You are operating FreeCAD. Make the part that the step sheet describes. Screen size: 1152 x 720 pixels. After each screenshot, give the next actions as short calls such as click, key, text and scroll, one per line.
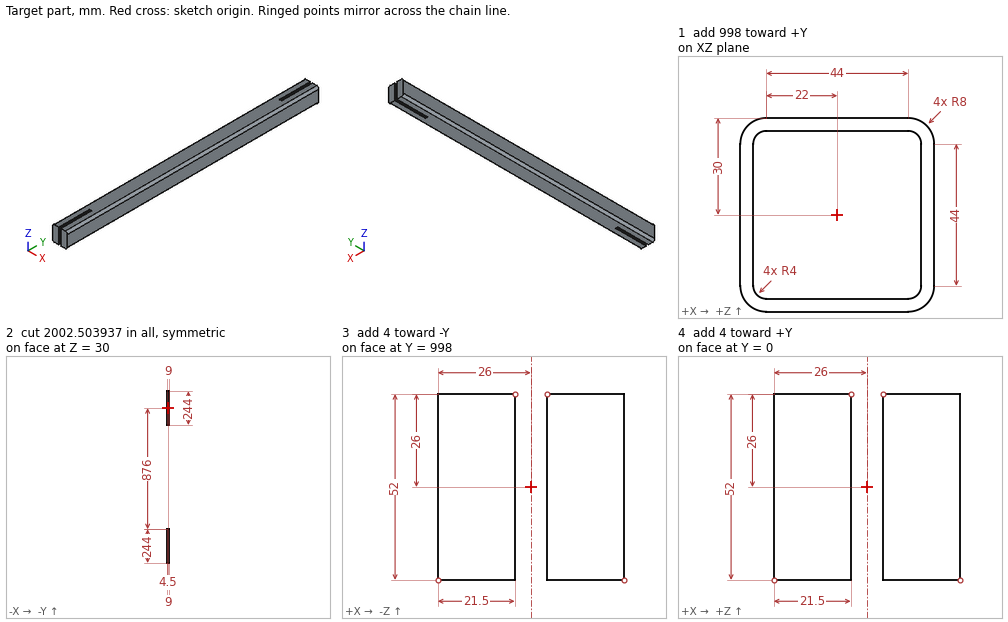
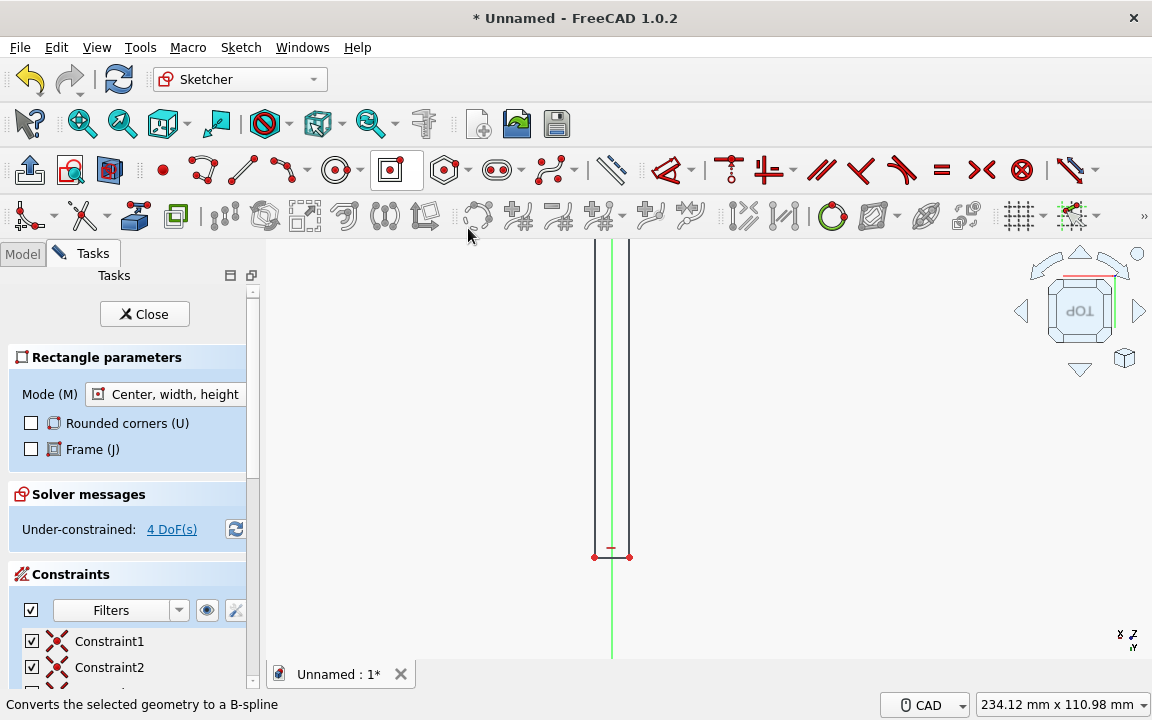
scroll(642, 566, down, 15)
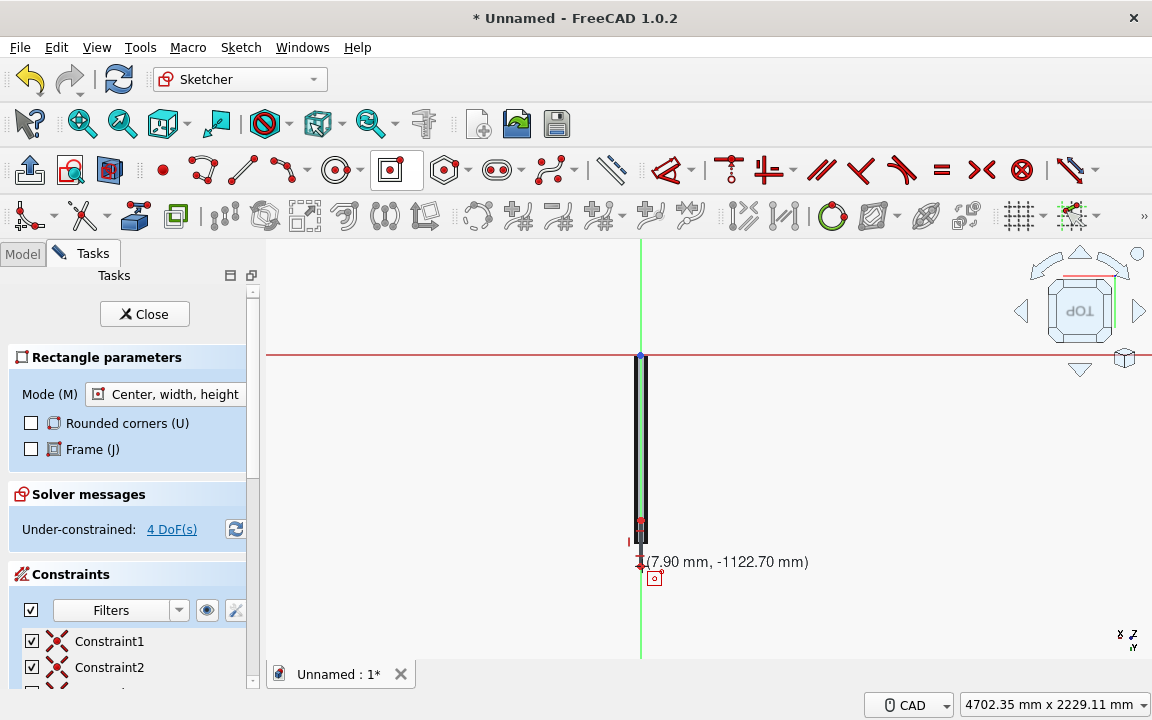
scroll(641, 355, up, 15)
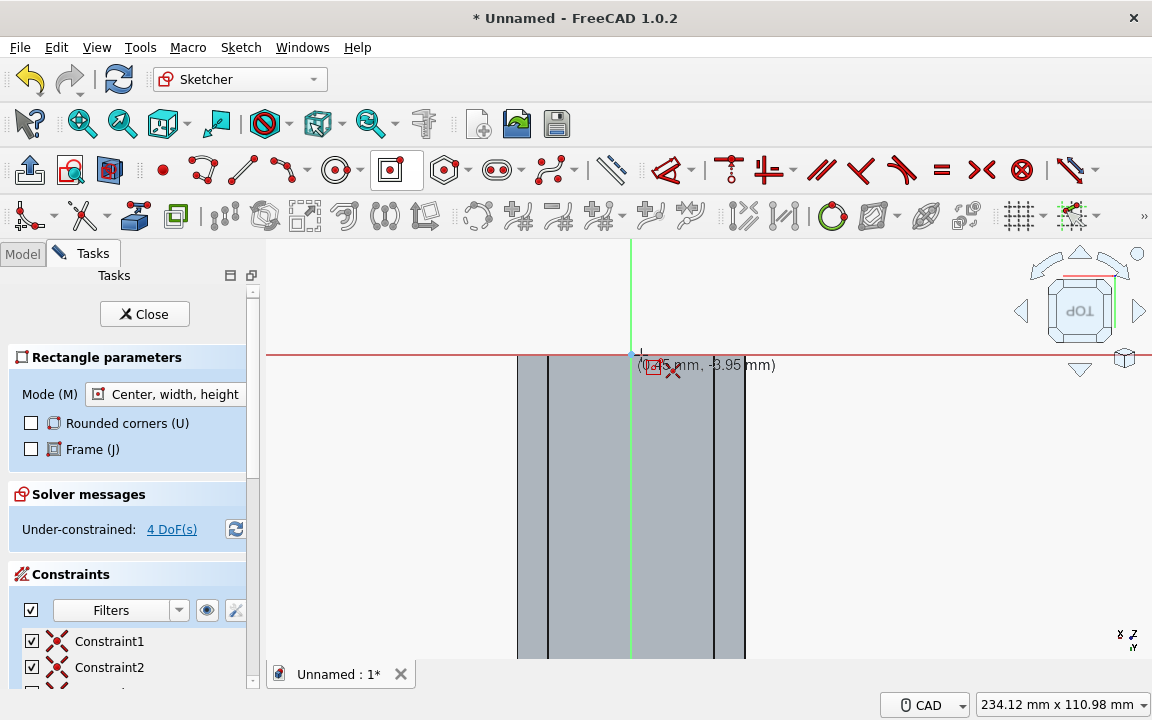
scroll(641, 355, down, 15)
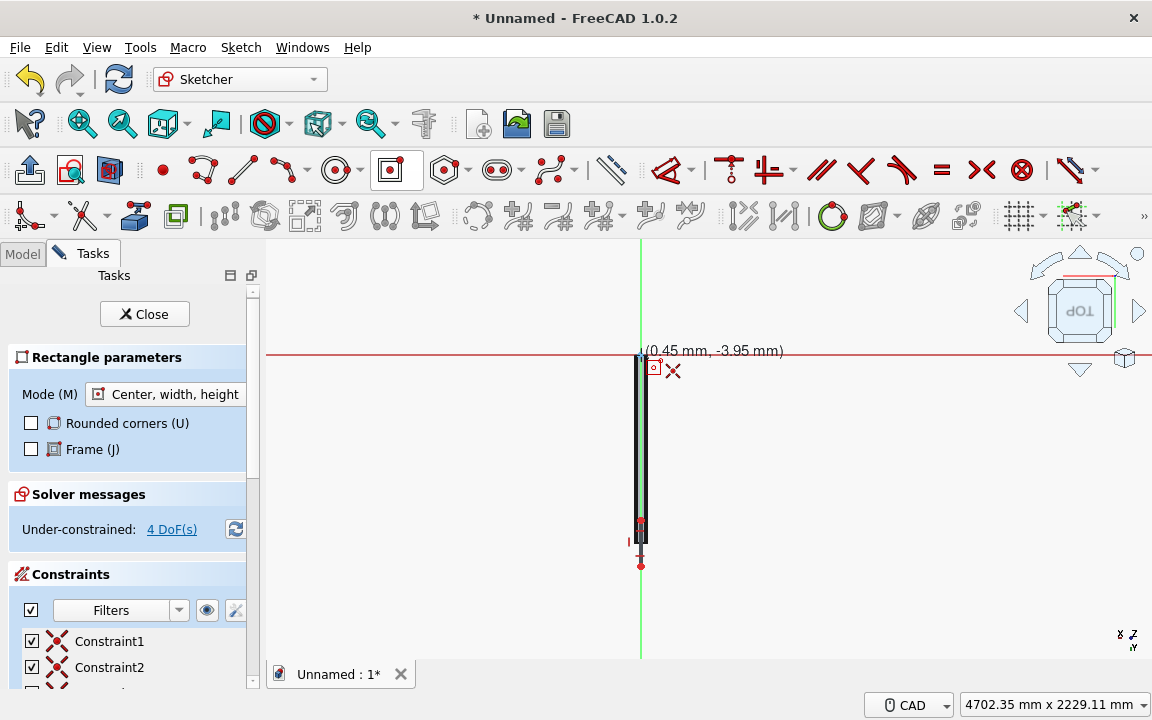
click(641, 355)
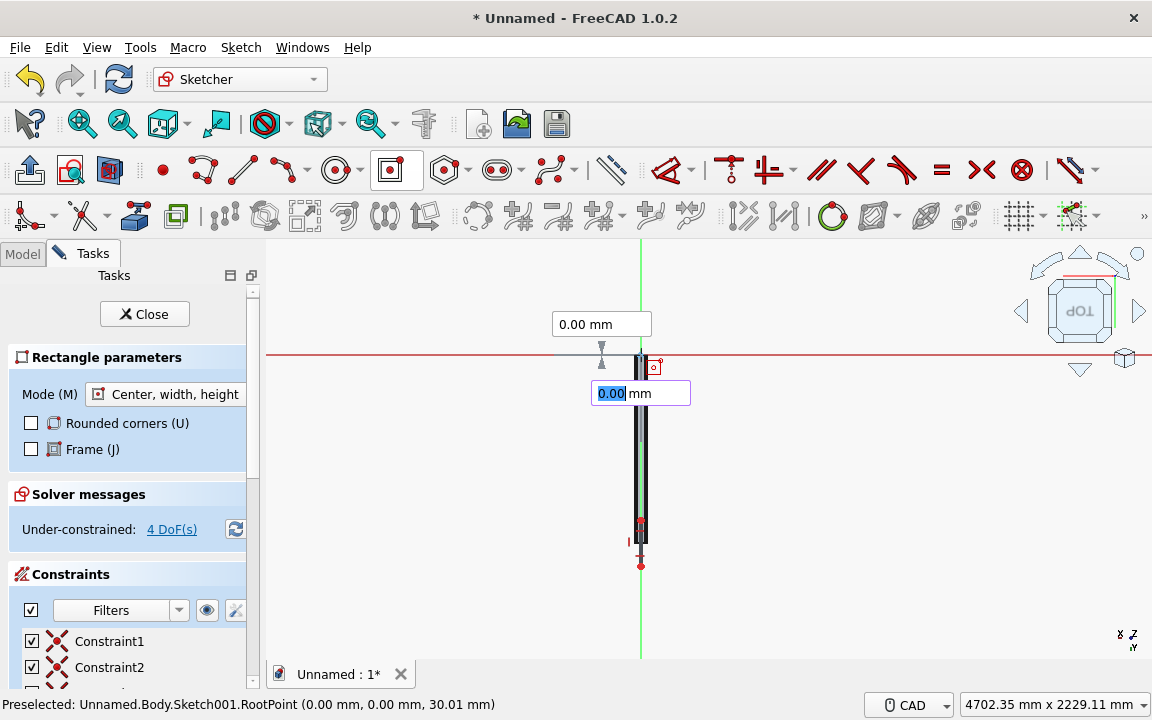
scroll(642, 332, up, 15)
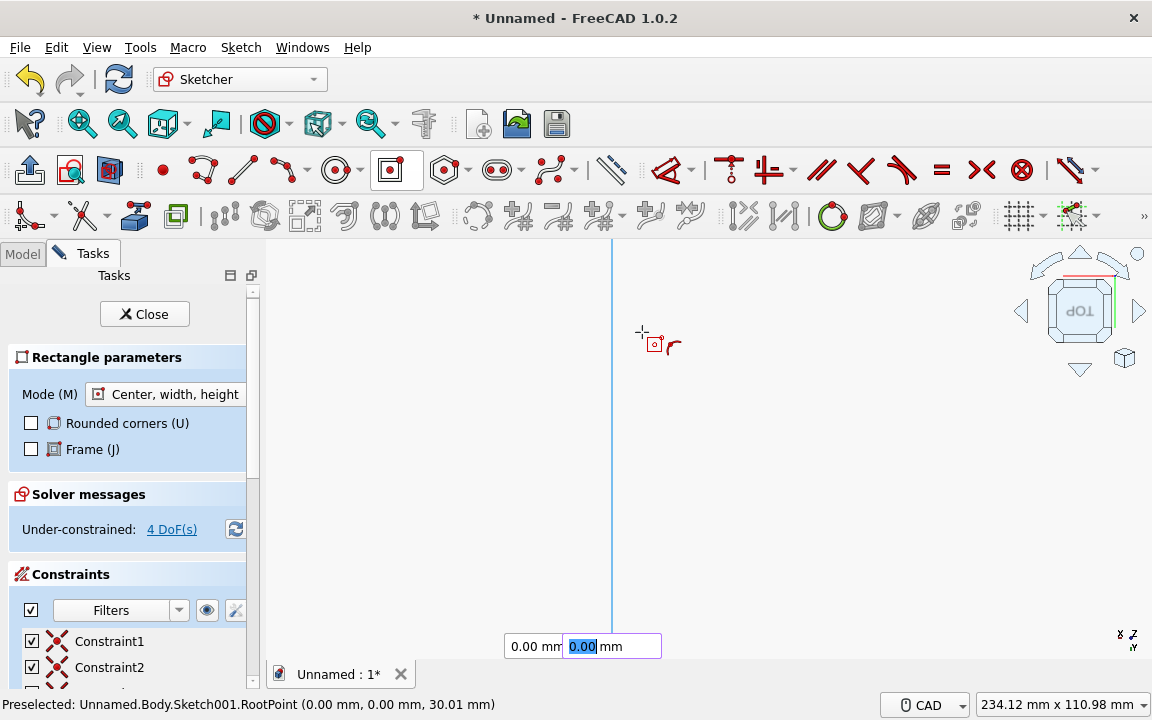
click(629, 333)
key(Escape)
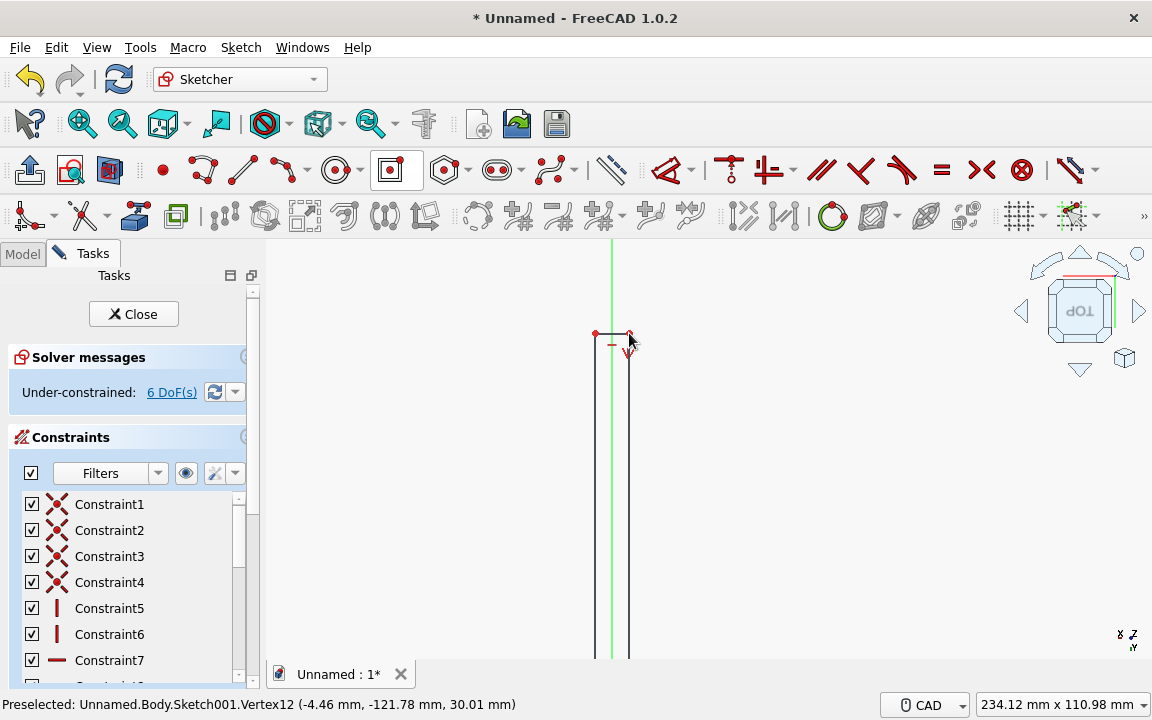
click(666, 170)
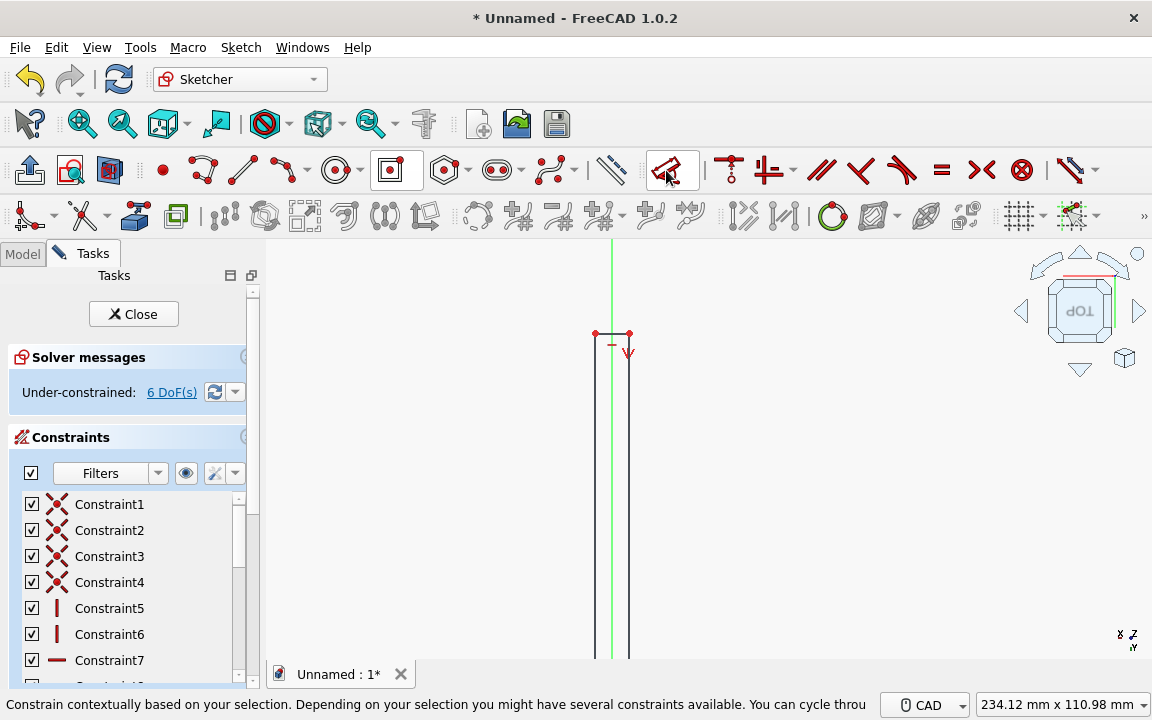
scroll(642, 332, down, 15)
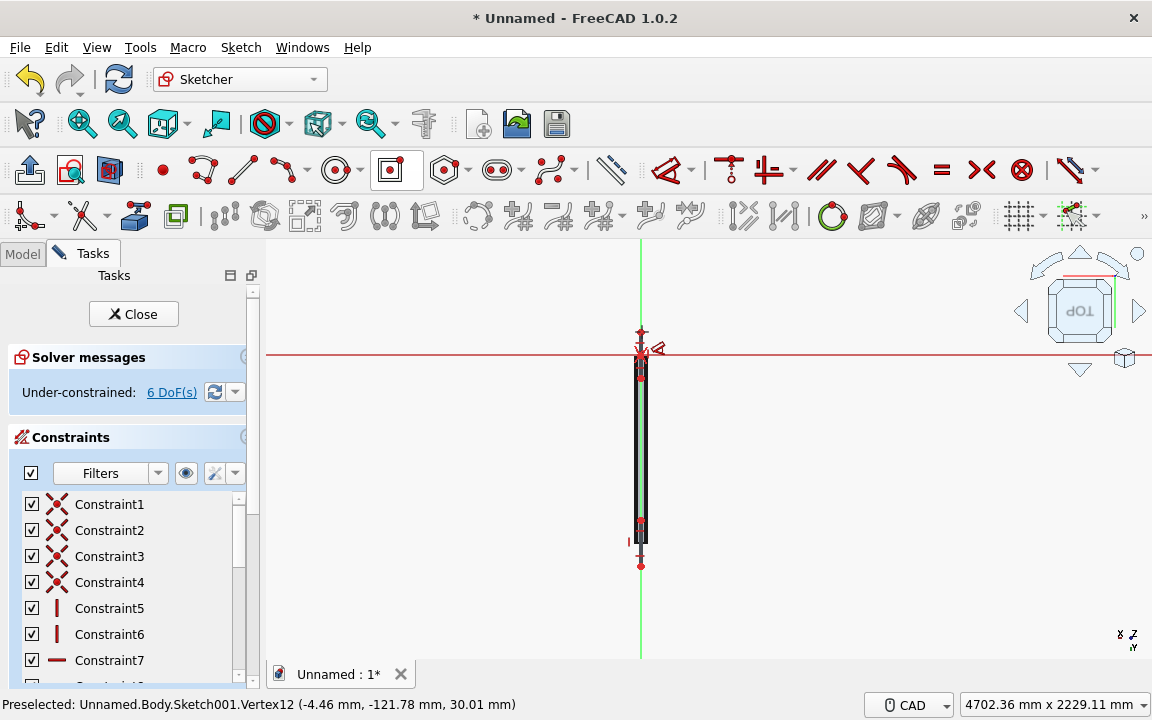
scroll(641, 566, up, 16)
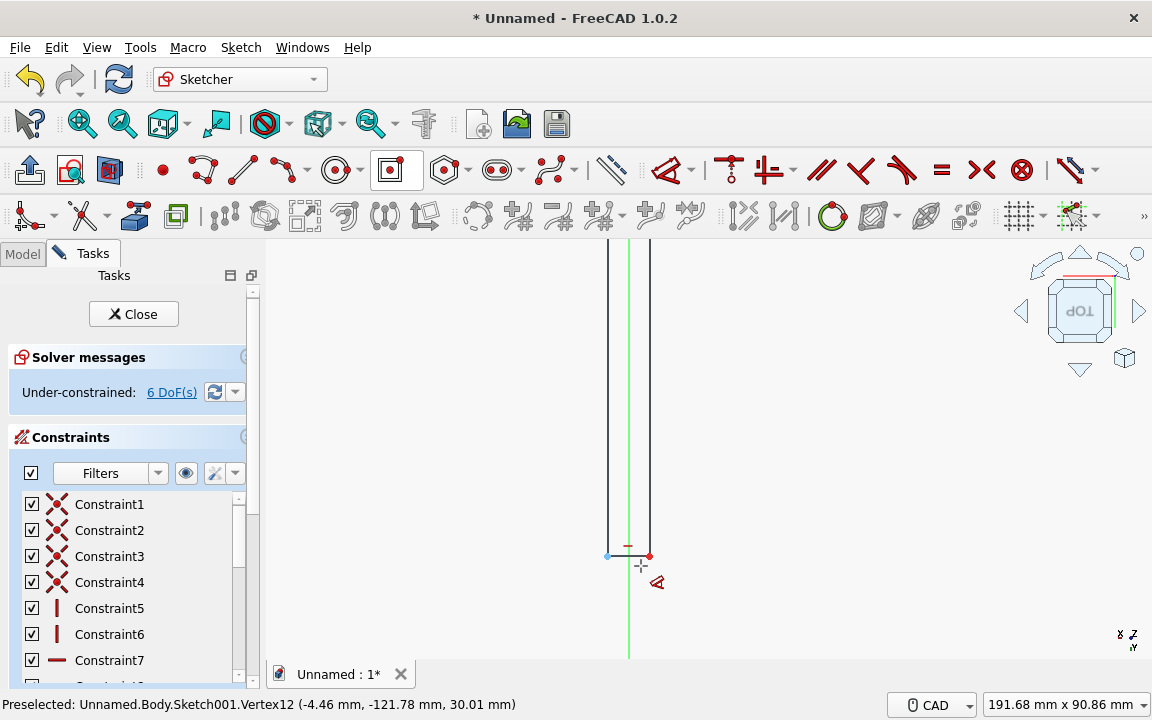
click(625, 556)
click(614, 590)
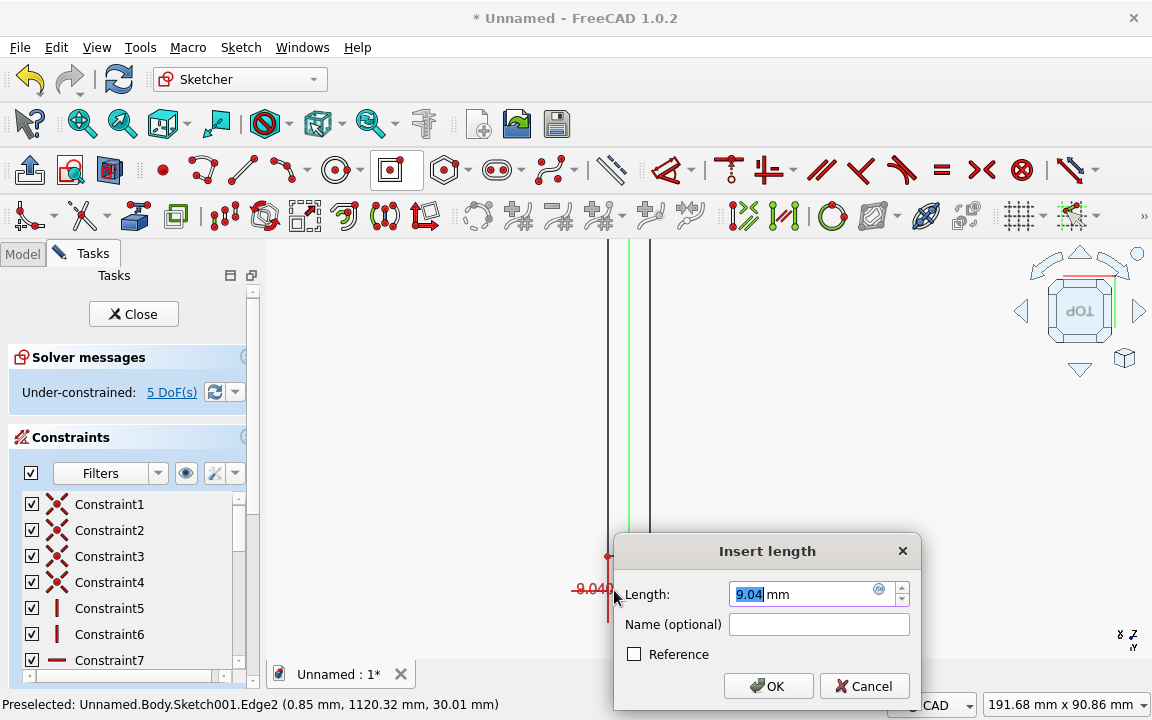
text(9)
key(Return)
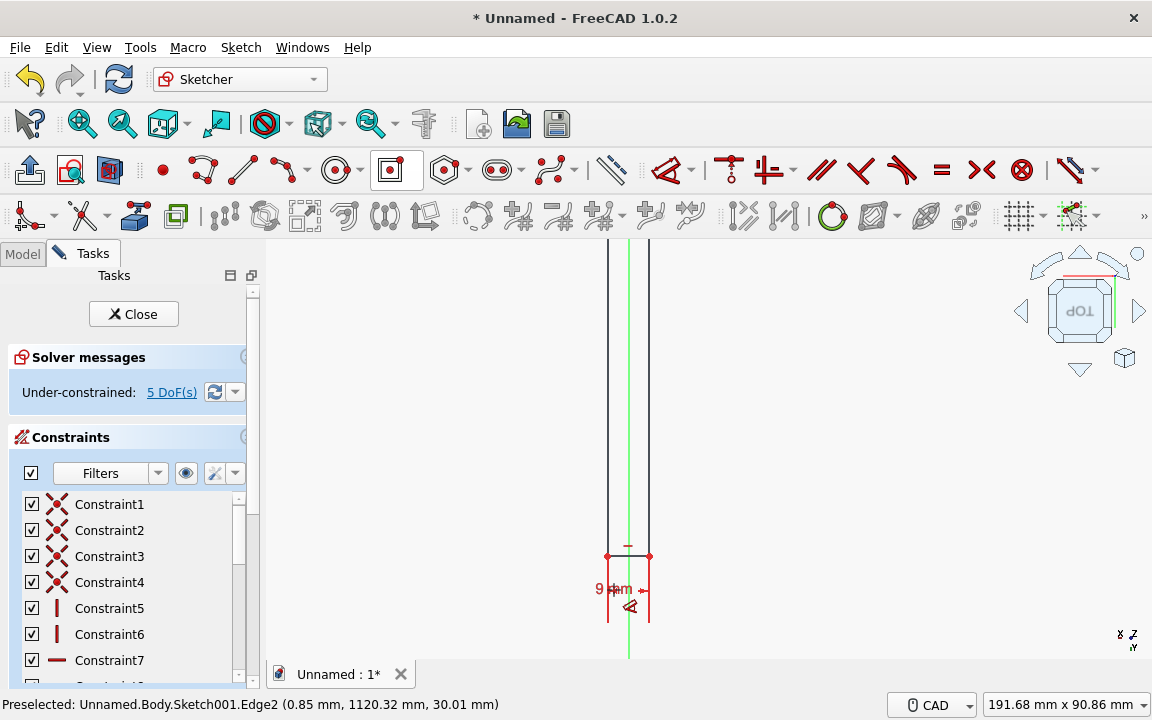
scroll(641, 594, down, 15)